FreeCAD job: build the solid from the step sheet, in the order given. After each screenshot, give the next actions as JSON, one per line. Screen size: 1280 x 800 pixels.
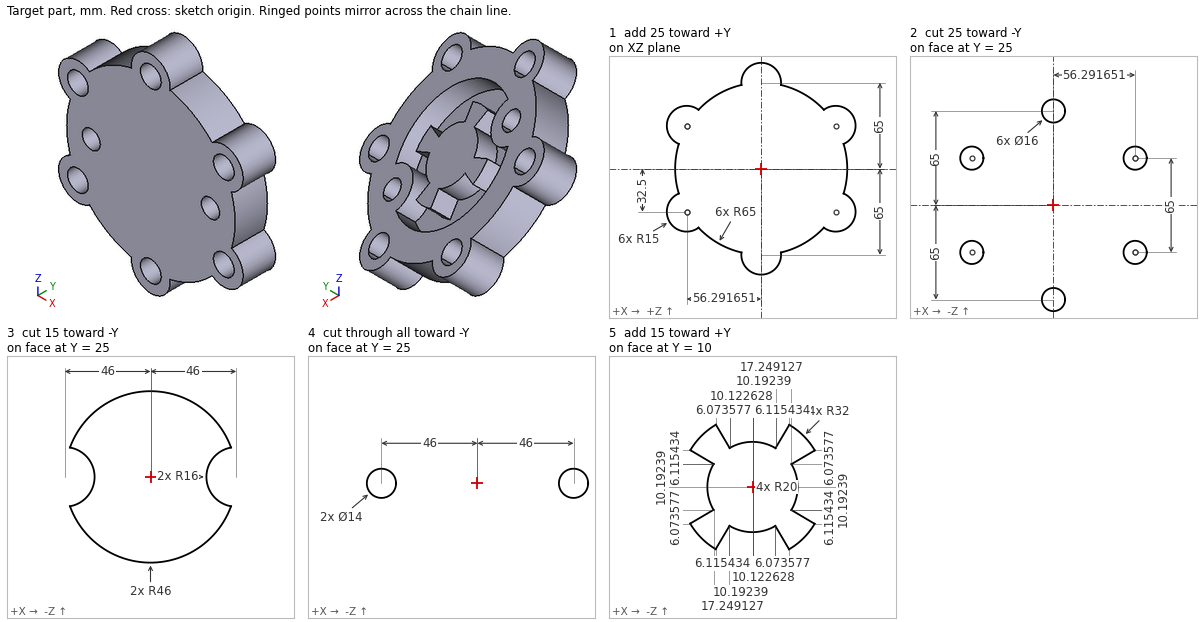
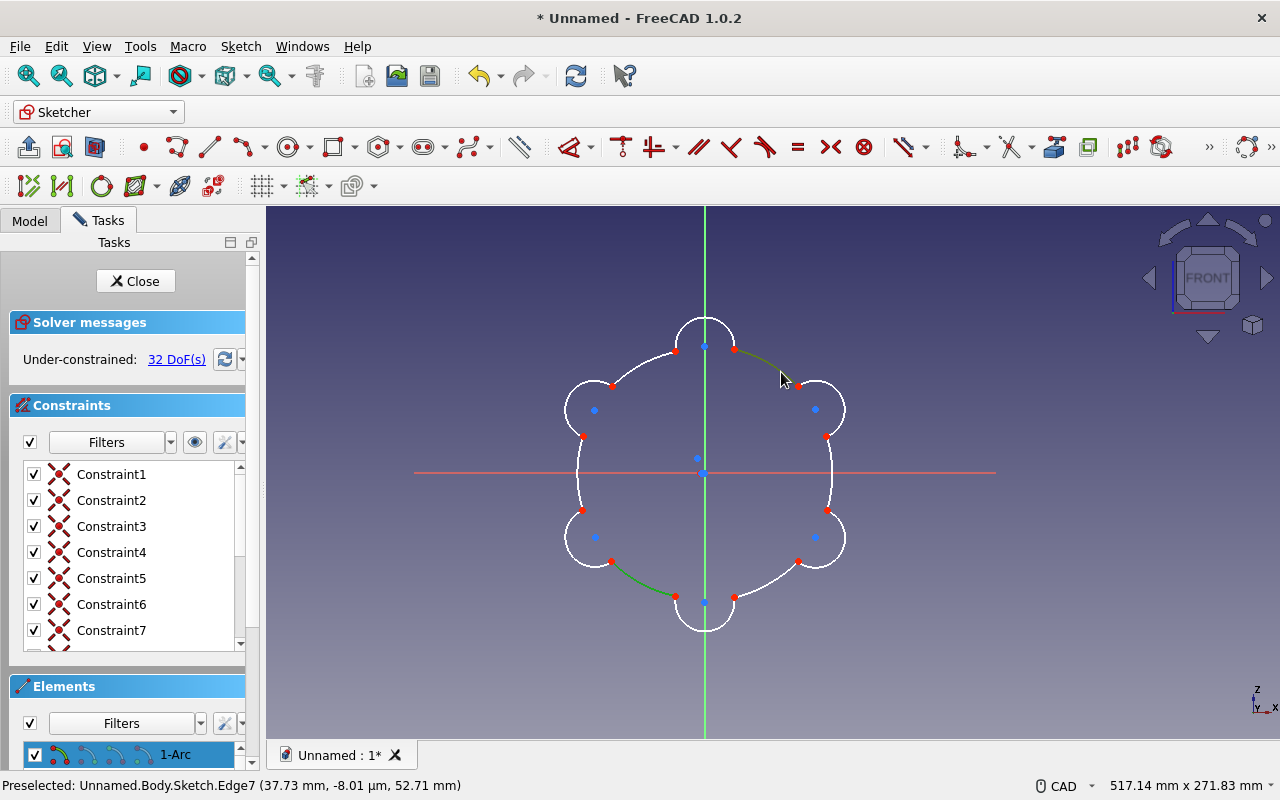
{"action": "left_click", "coordinate": [621, 148]}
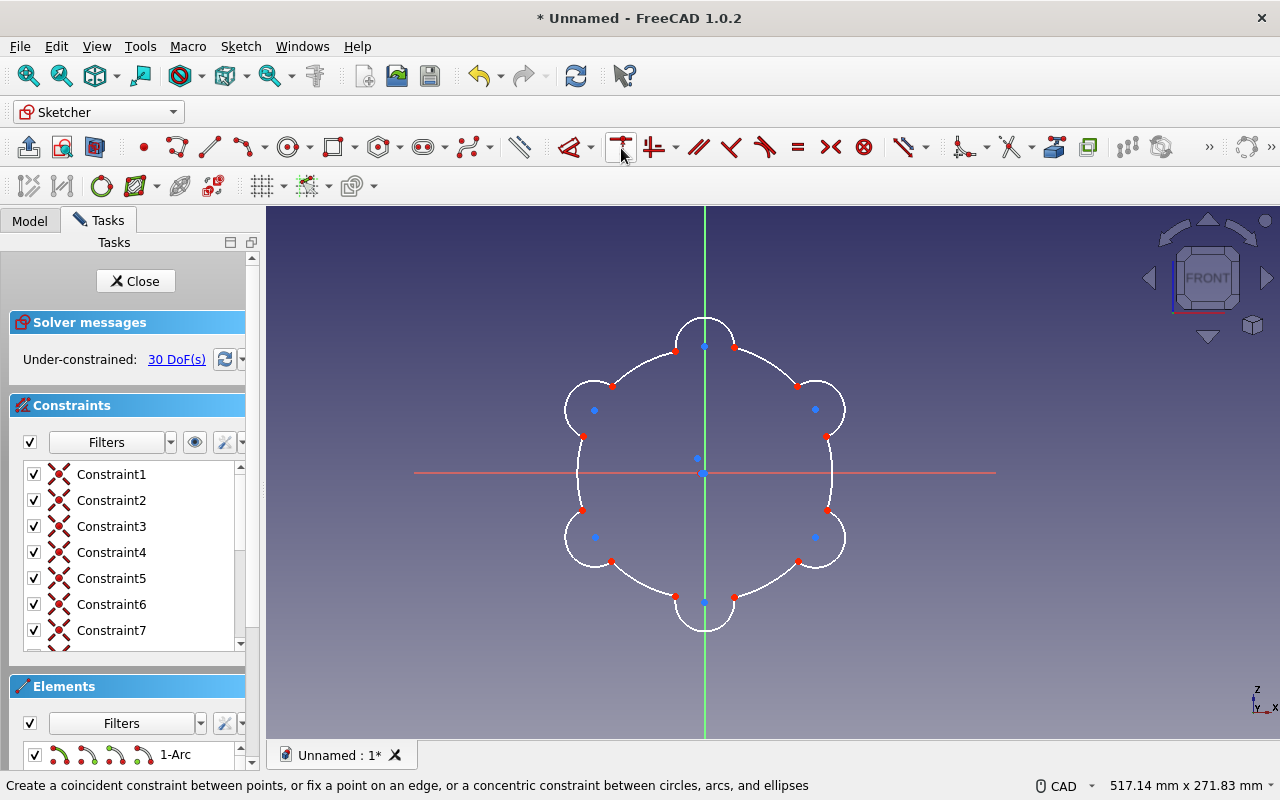
{"action": "left_click", "coordinate": [629, 576]}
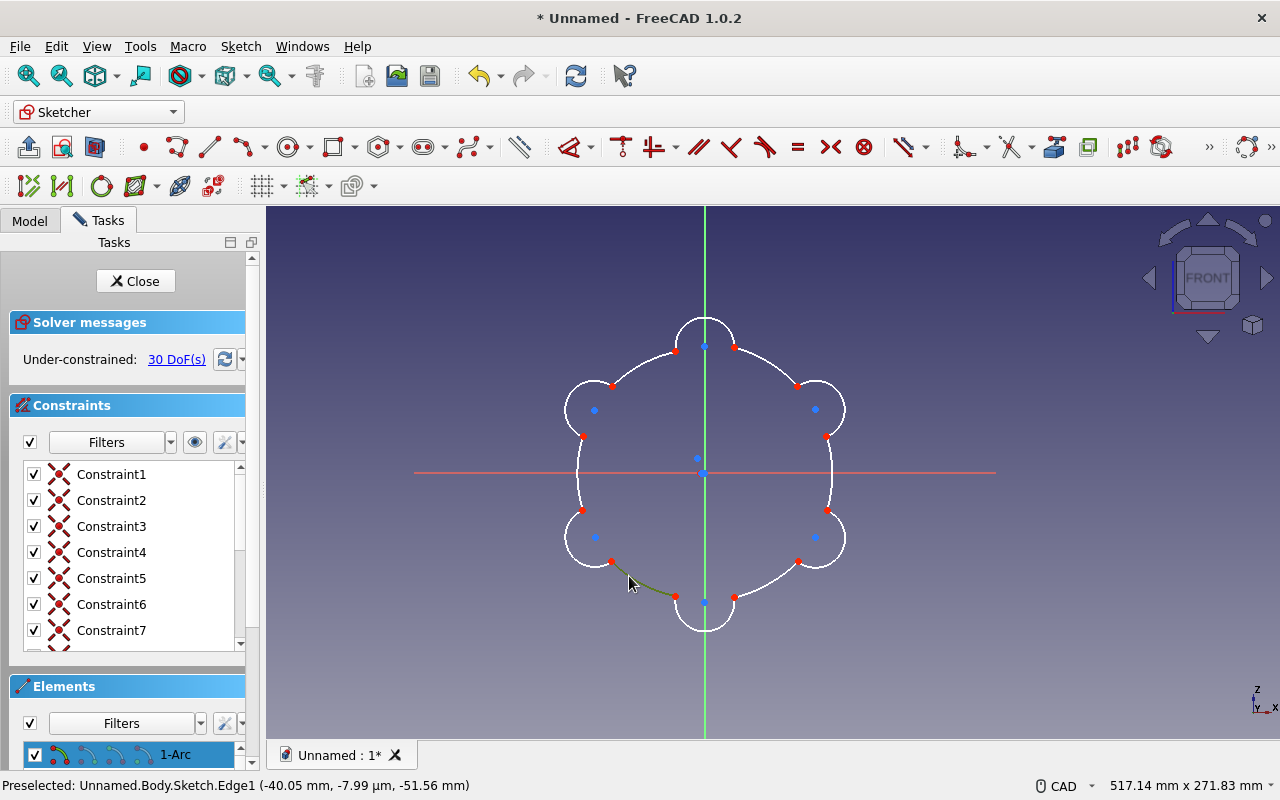
{"action": "left_click", "coordinate": [831, 489]}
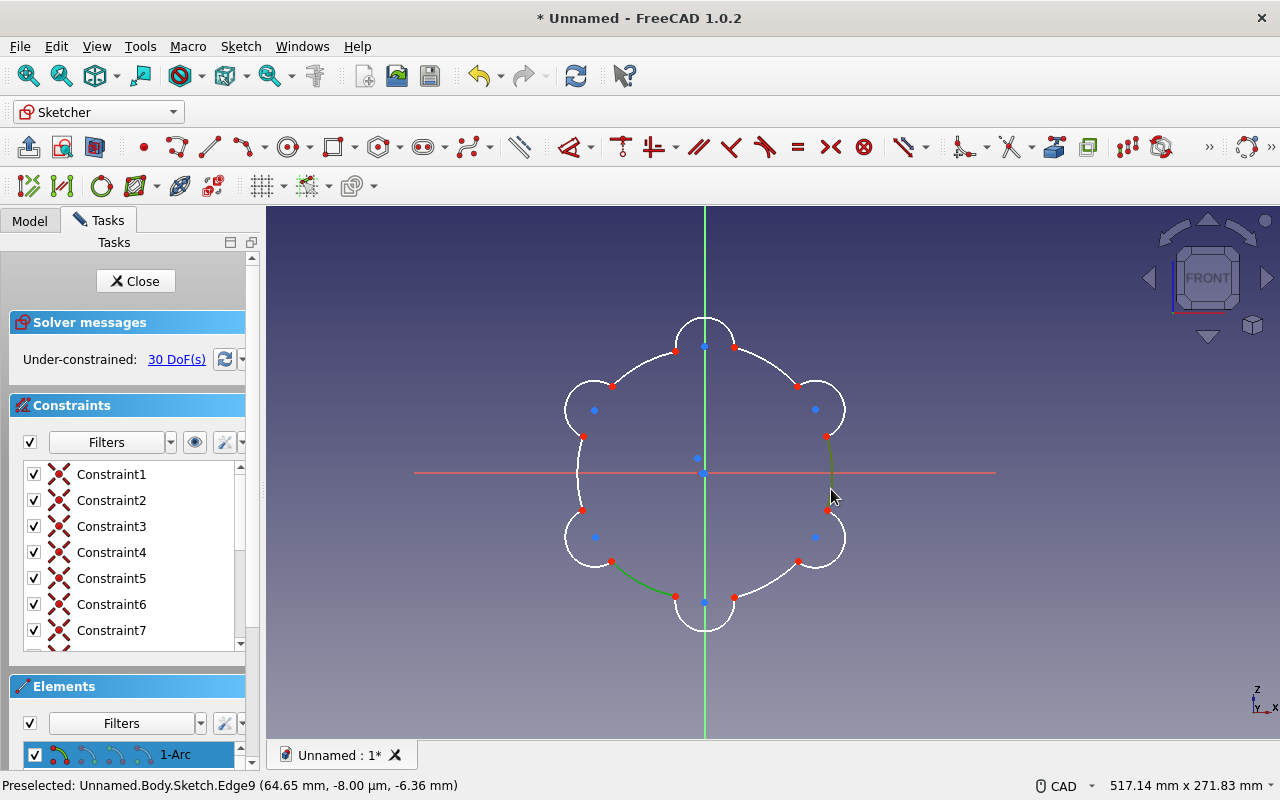
{"action": "left_click", "coordinate": [621, 148]}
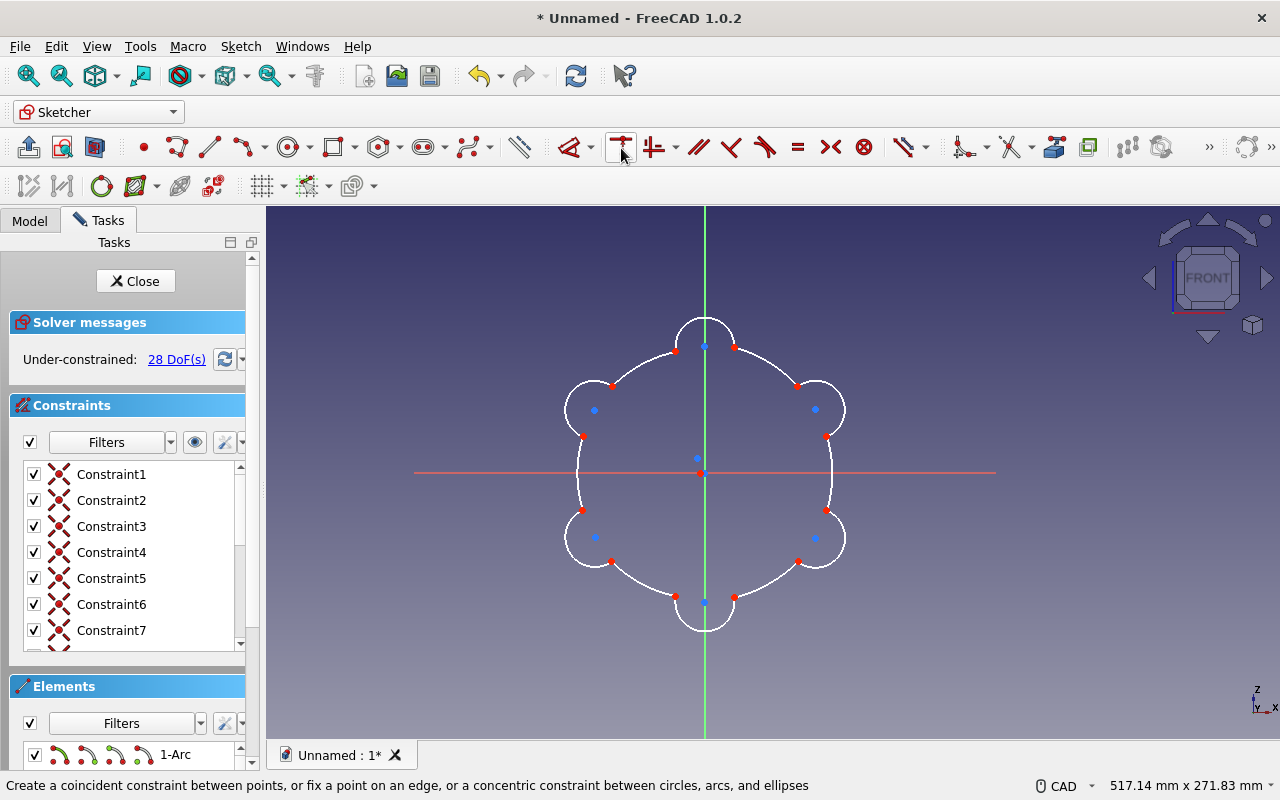
{"action": "left_click", "coordinate": [629, 576]}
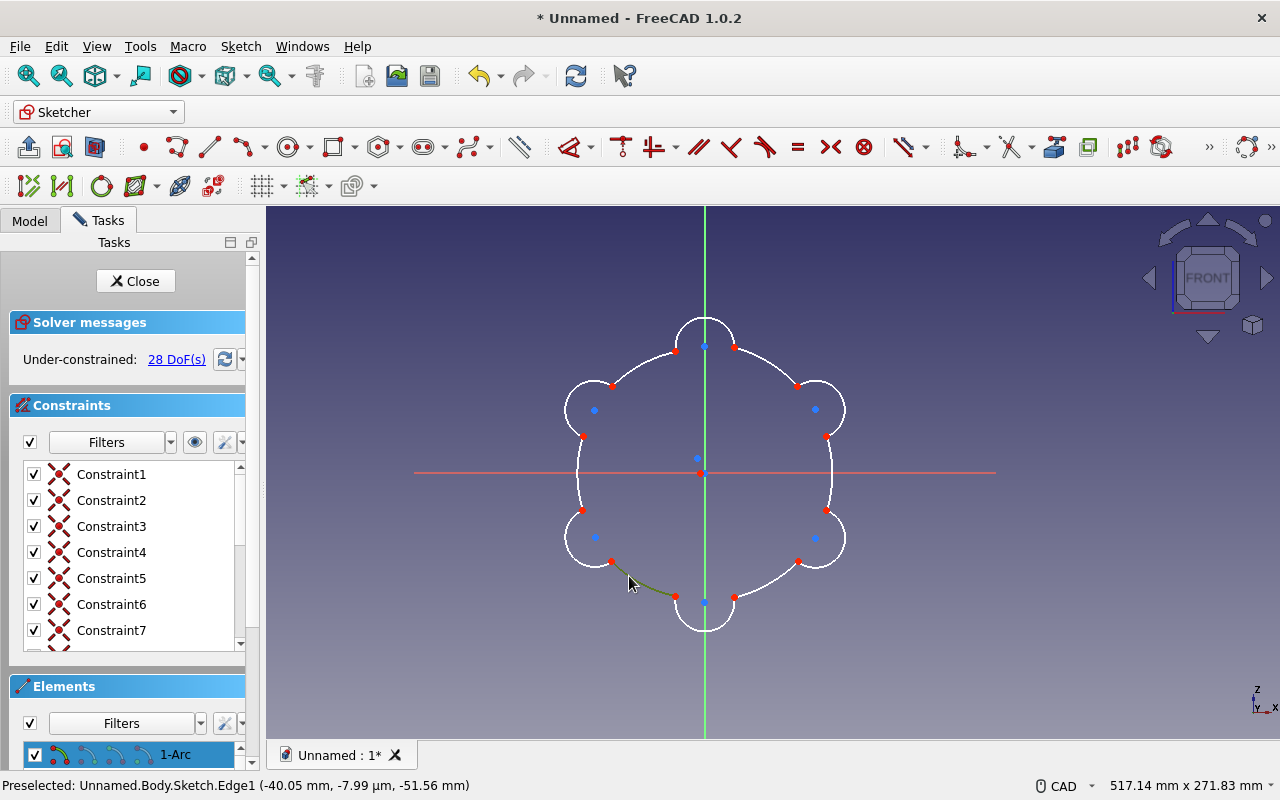
{"action": "left_click", "coordinate": [755, 591]}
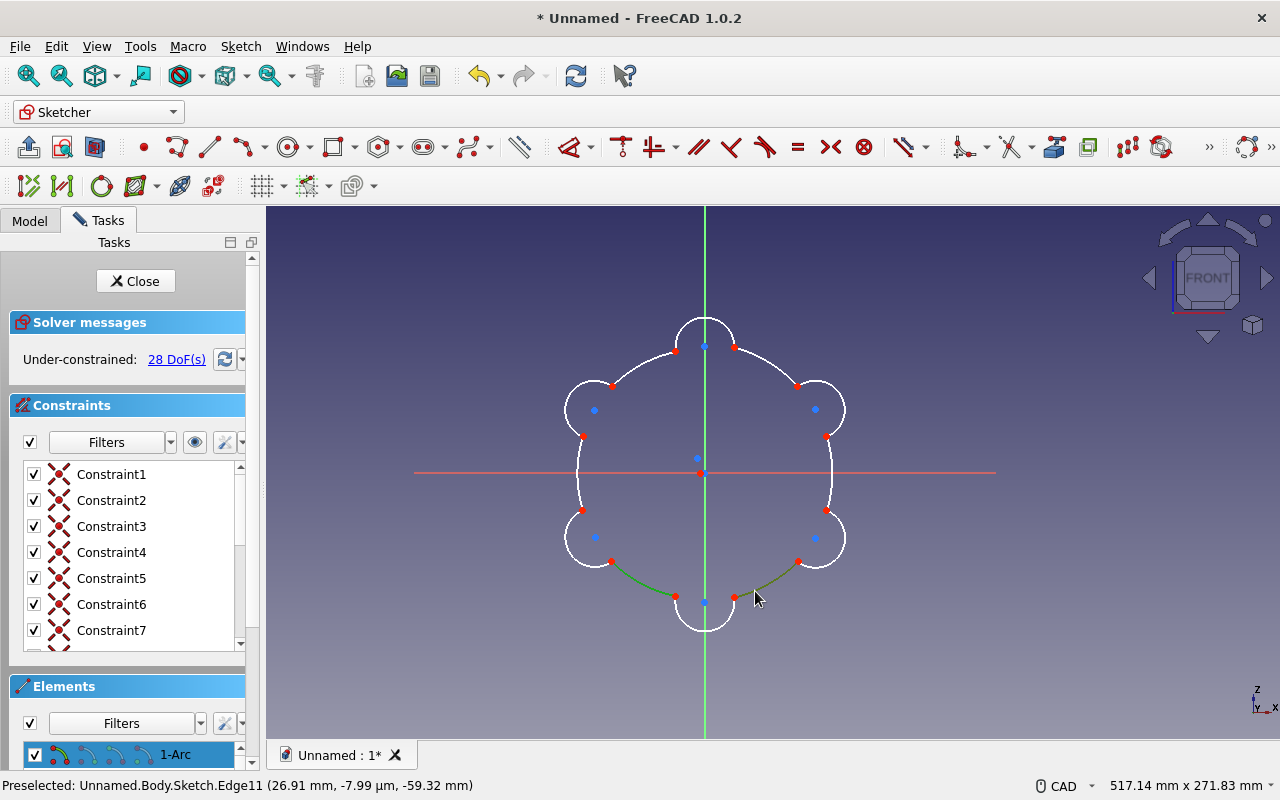
{"action": "left_click", "coordinate": [621, 148]}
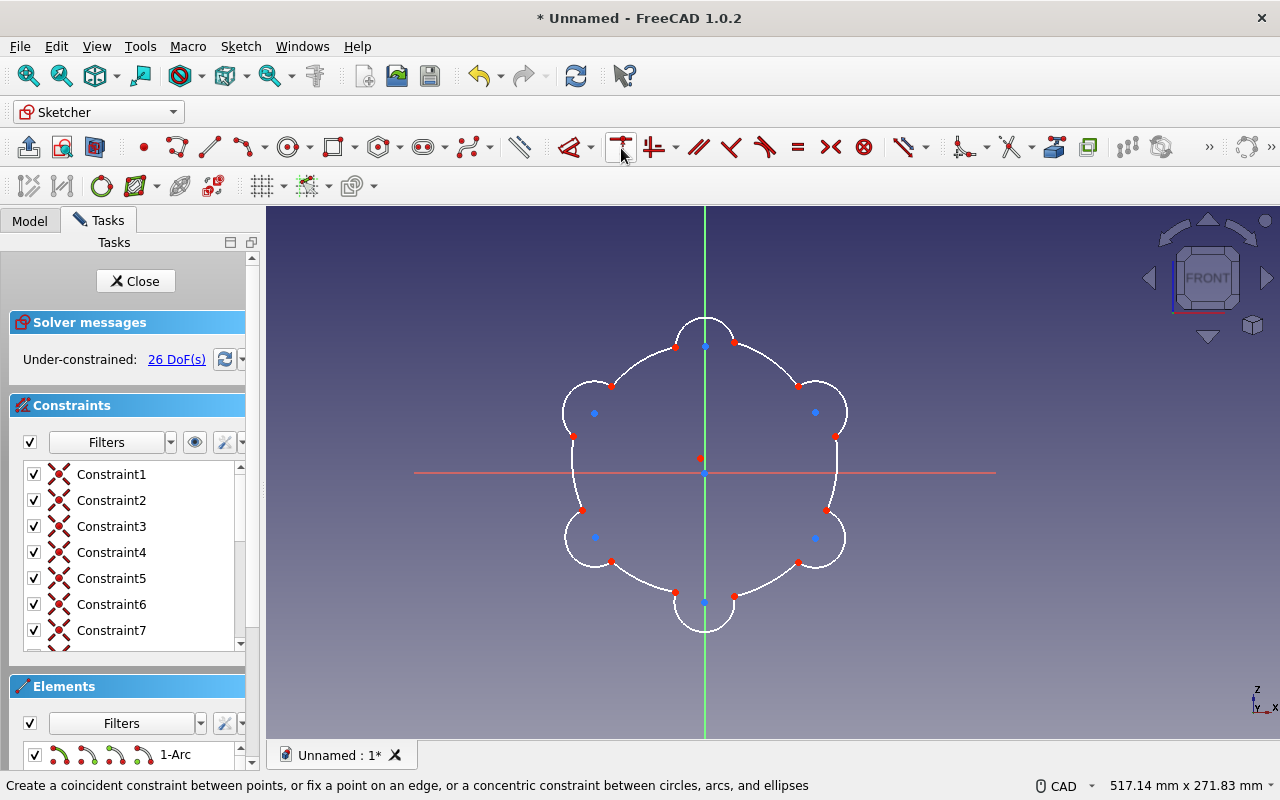
{"action": "scroll", "coordinate": [703, 466], "scroll_direction": "up", "scroll_amount": 2}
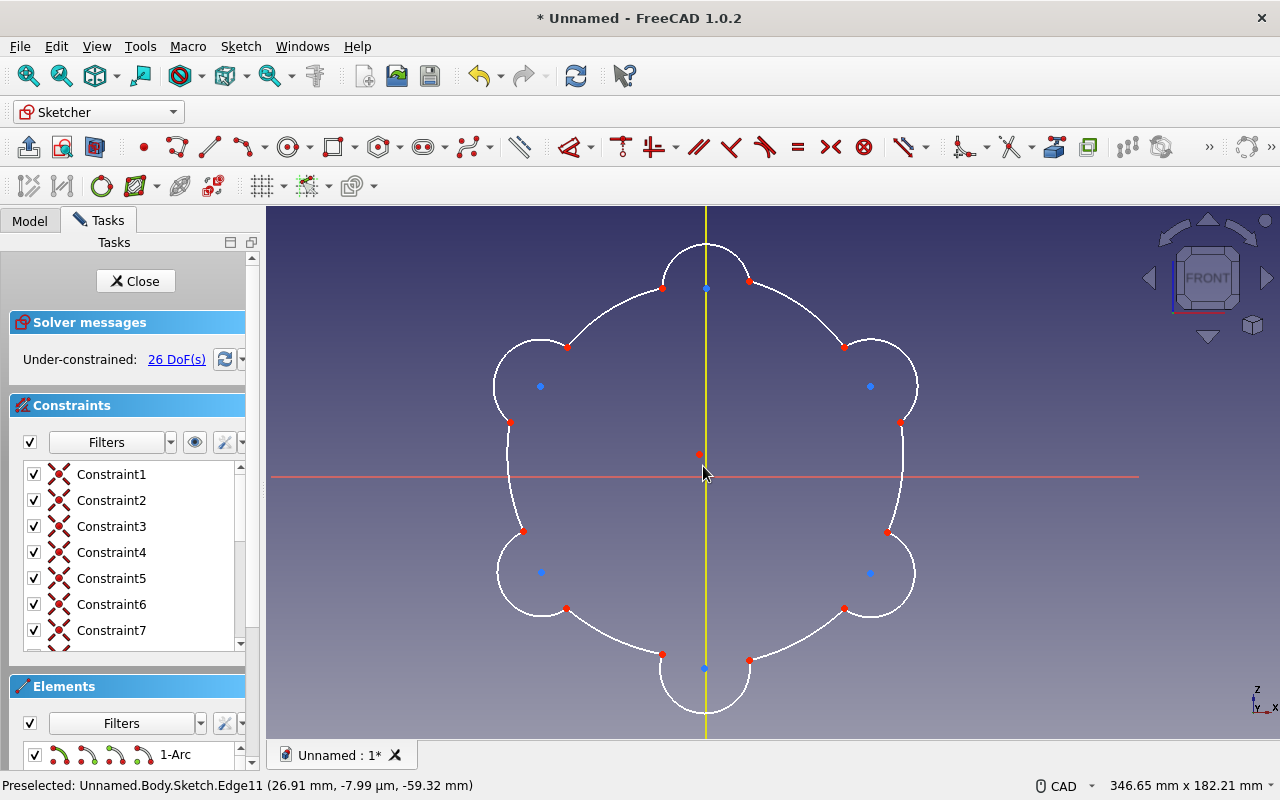
{"action": "left_click_drag", "start_coordinate": [689, 444], "coordinate": [716, 487]}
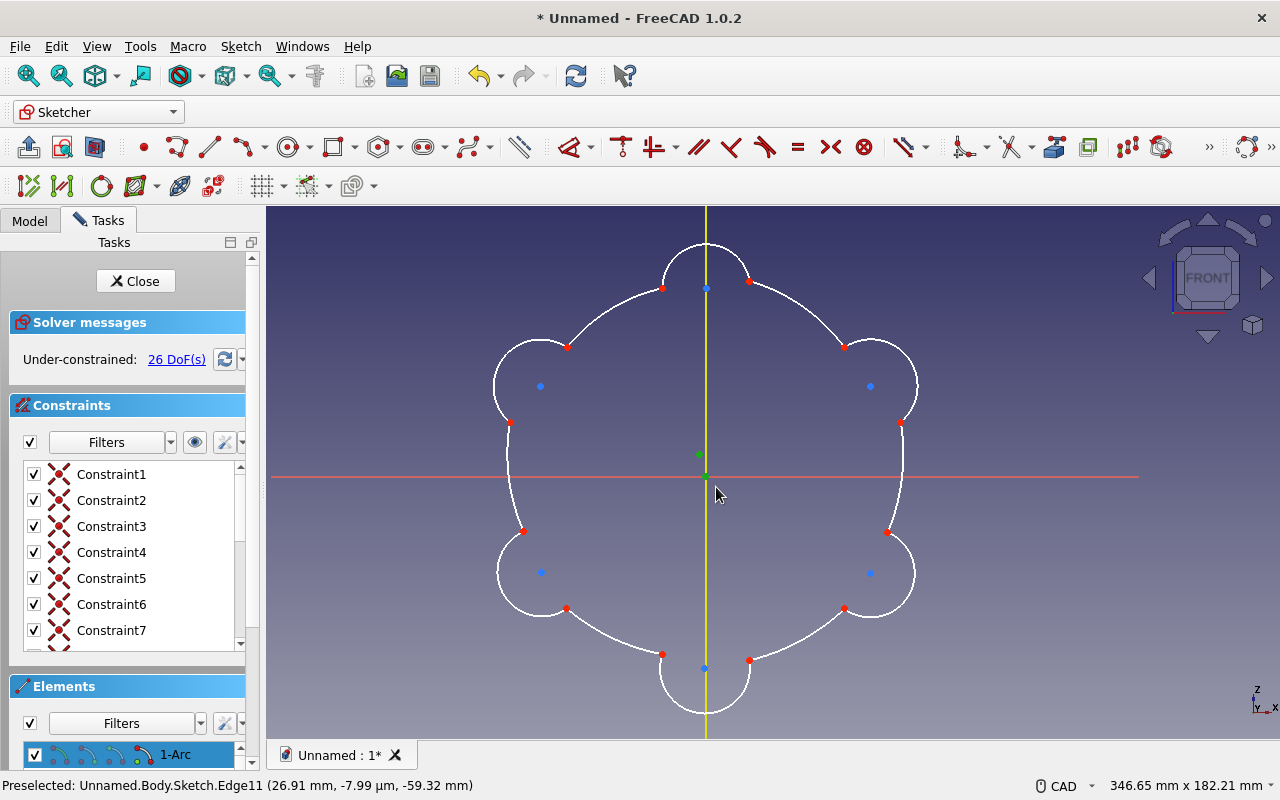
{"action": "left_click", "coordinate": [621, 148]}